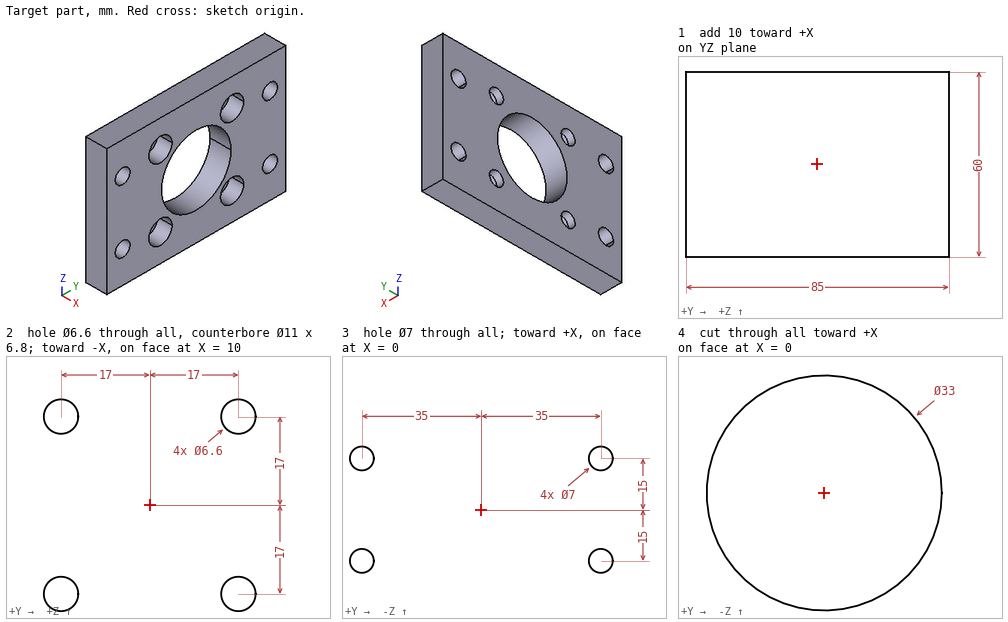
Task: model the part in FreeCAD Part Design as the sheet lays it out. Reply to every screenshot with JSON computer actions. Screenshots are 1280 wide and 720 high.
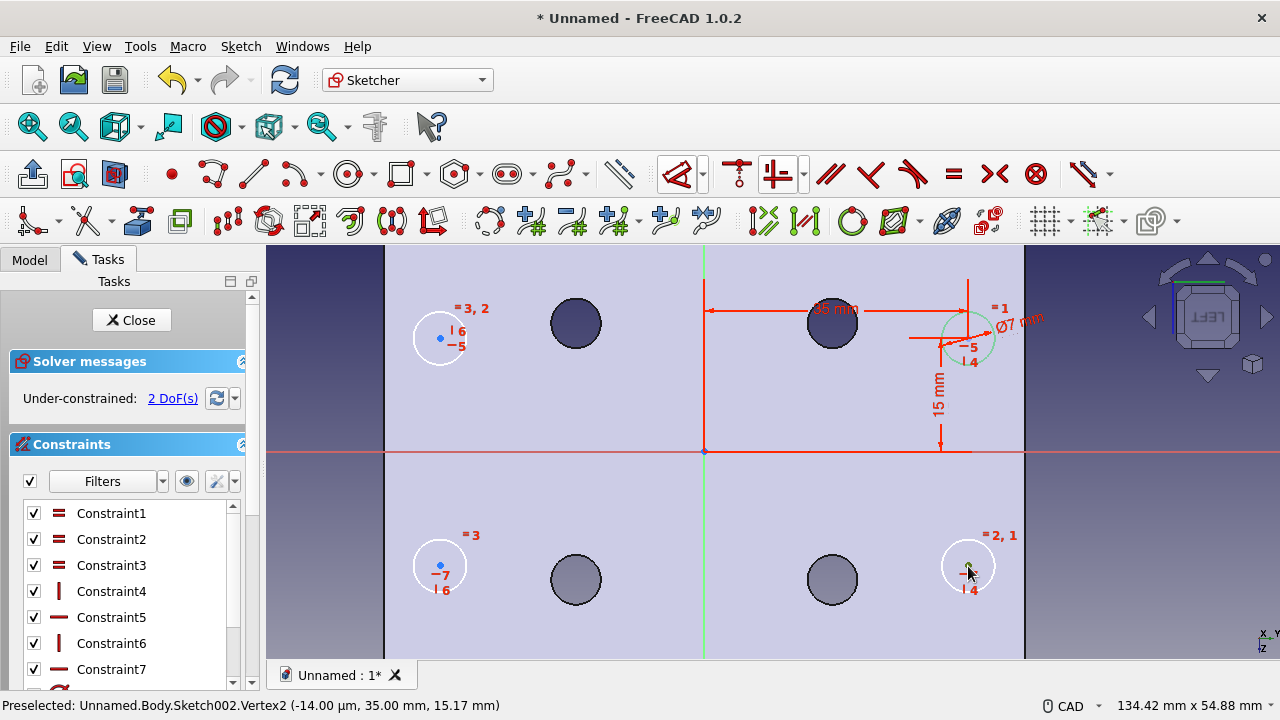
{"action": "key", "text": "i"}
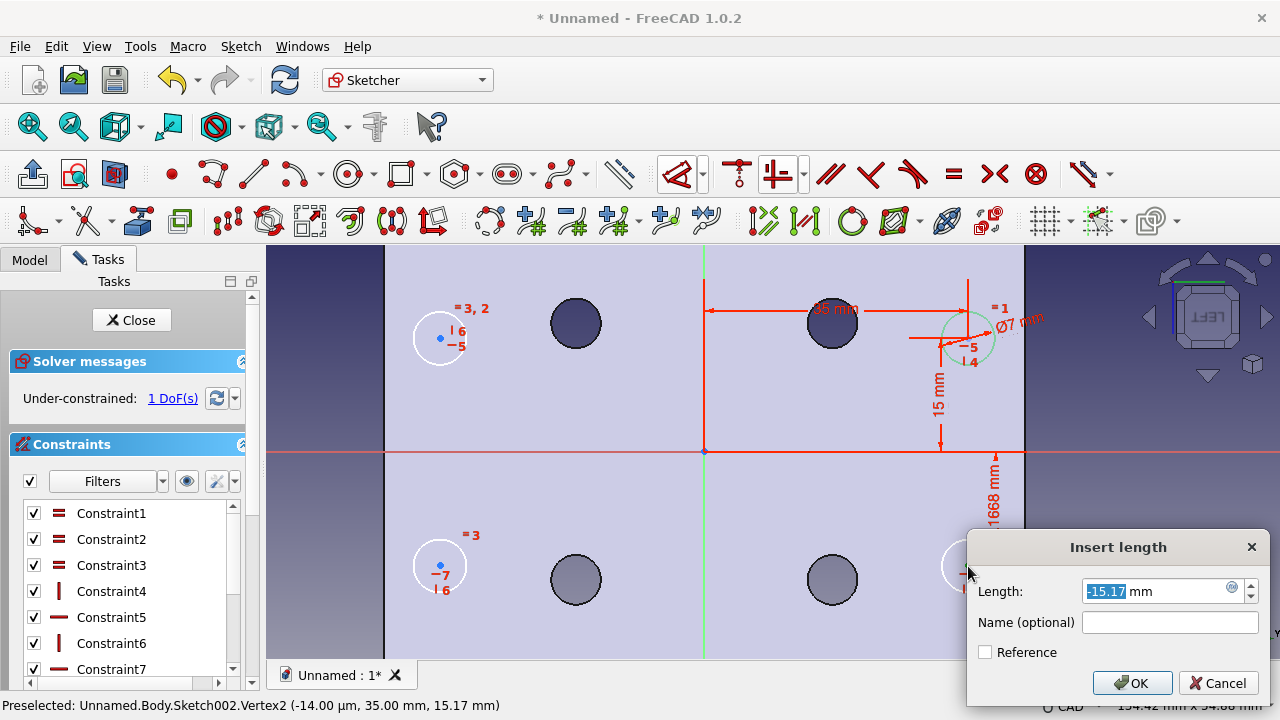
{"action": "type", "text": "-15"}
{"action": "key", "text": "Return"}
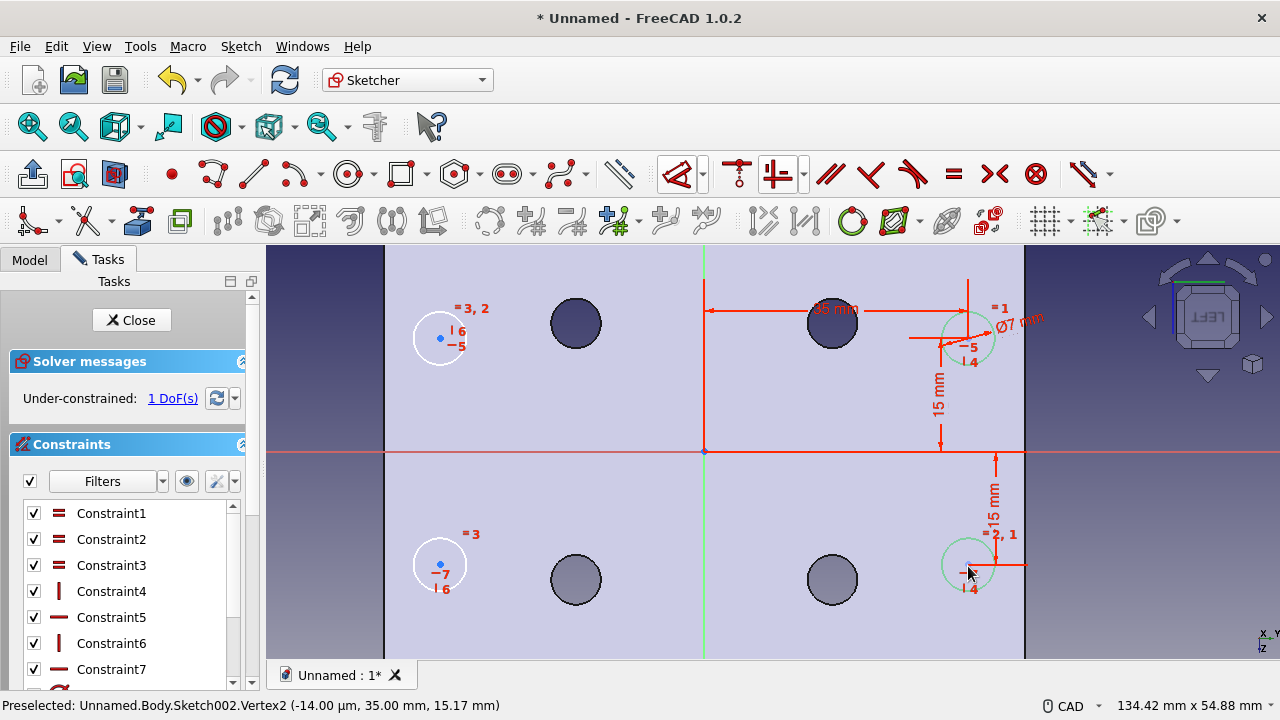
{"action": "left_click", "coordinate": [440, 338]}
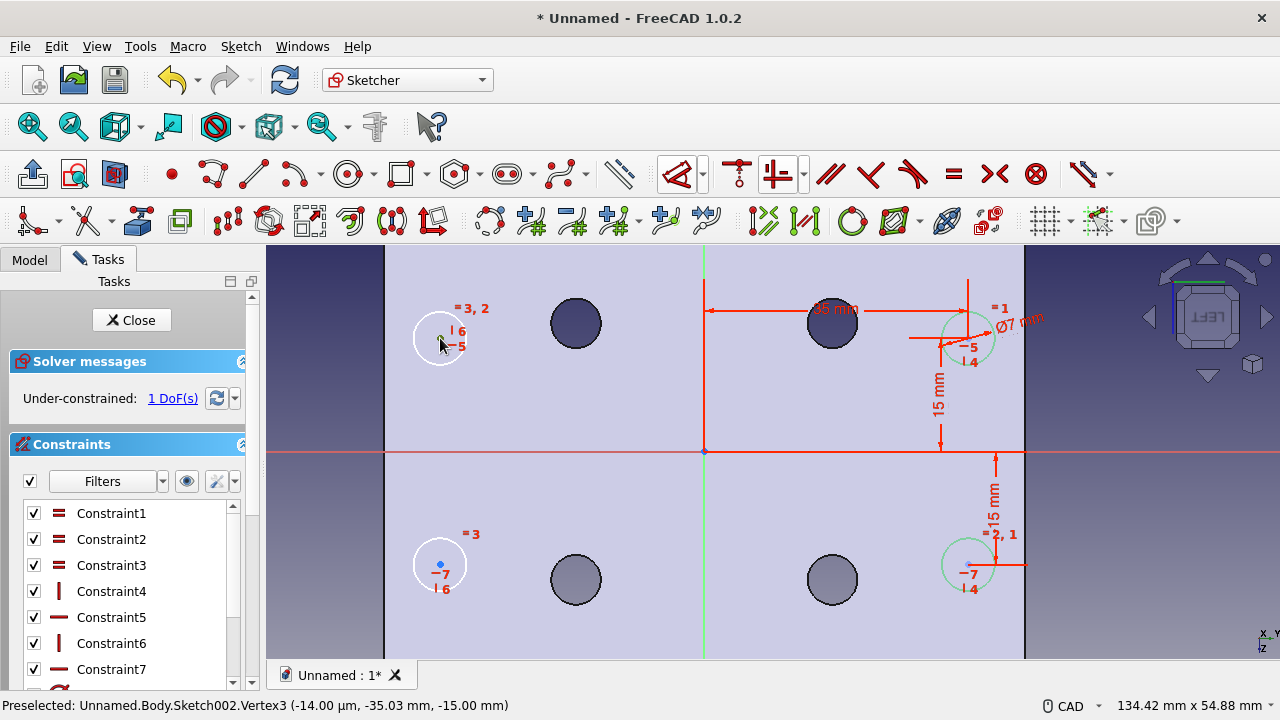
{"action": "key", "text": "l"}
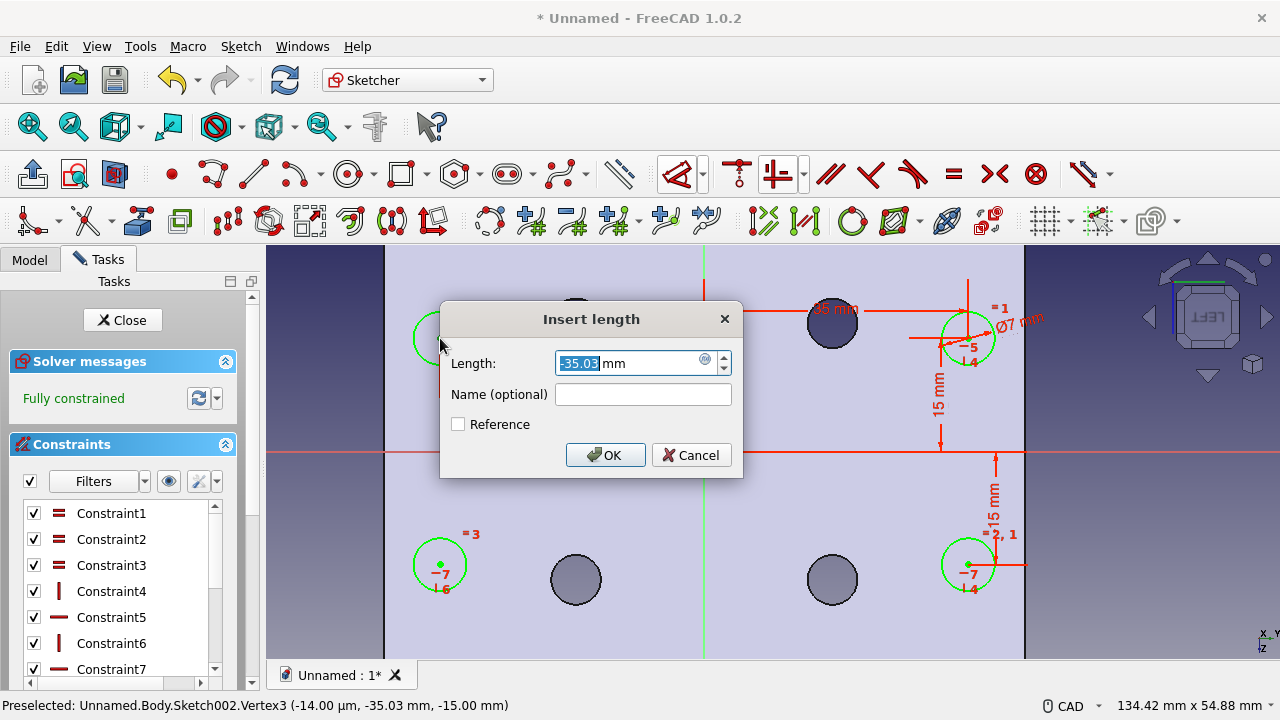
{"action": "type", "text": "-35"}
{"action": "key", "text": "Return"}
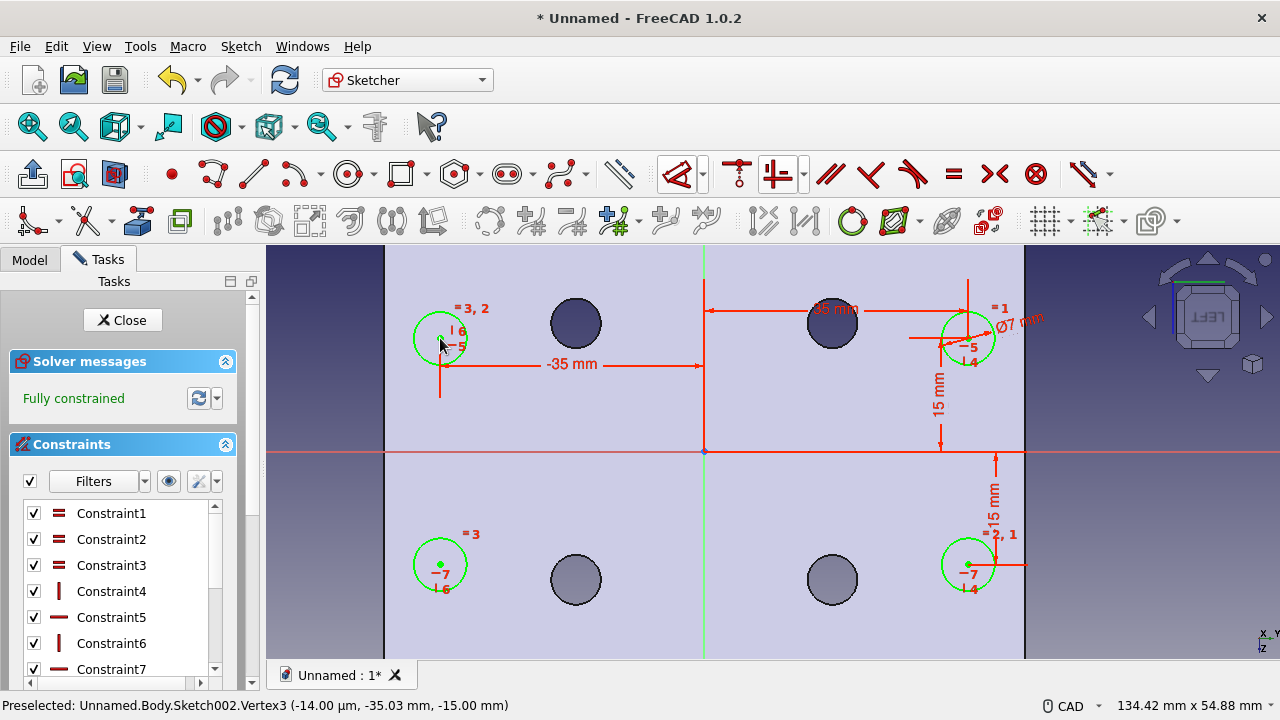
{"action": "left_click", "coordinate": [123, 320]}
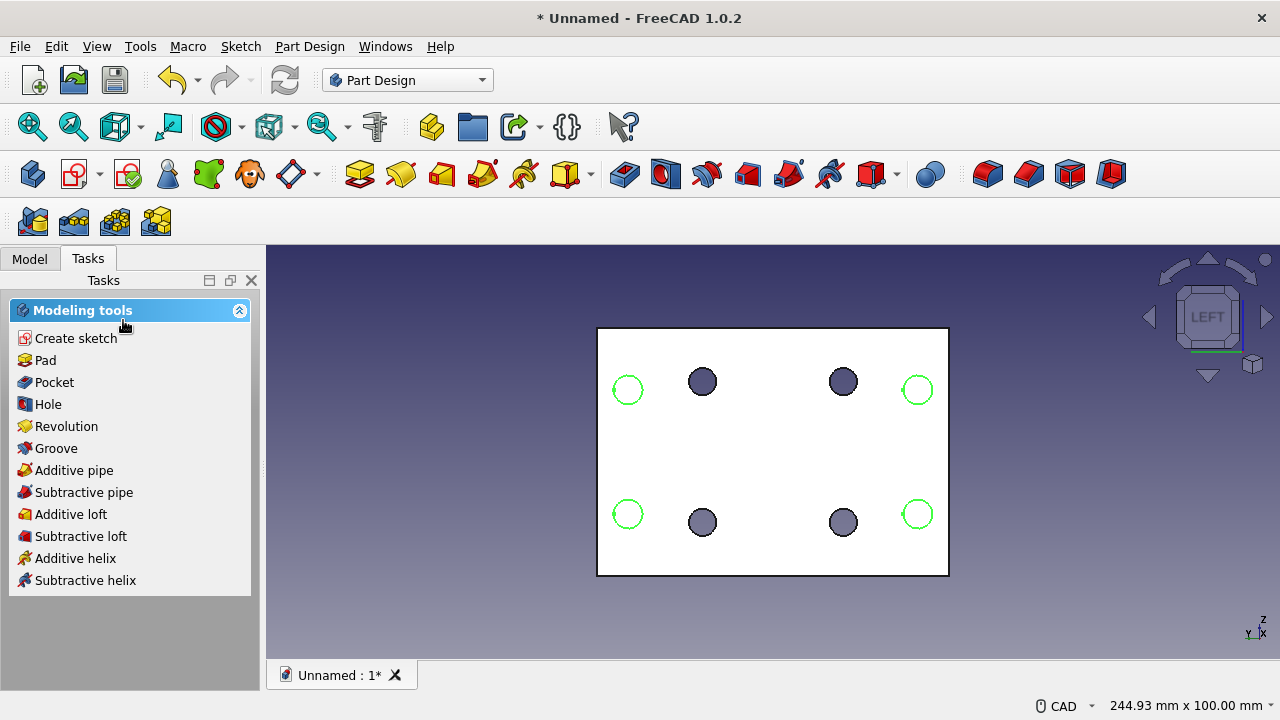
{"action": "left_click", "coordinate": [666, 174]}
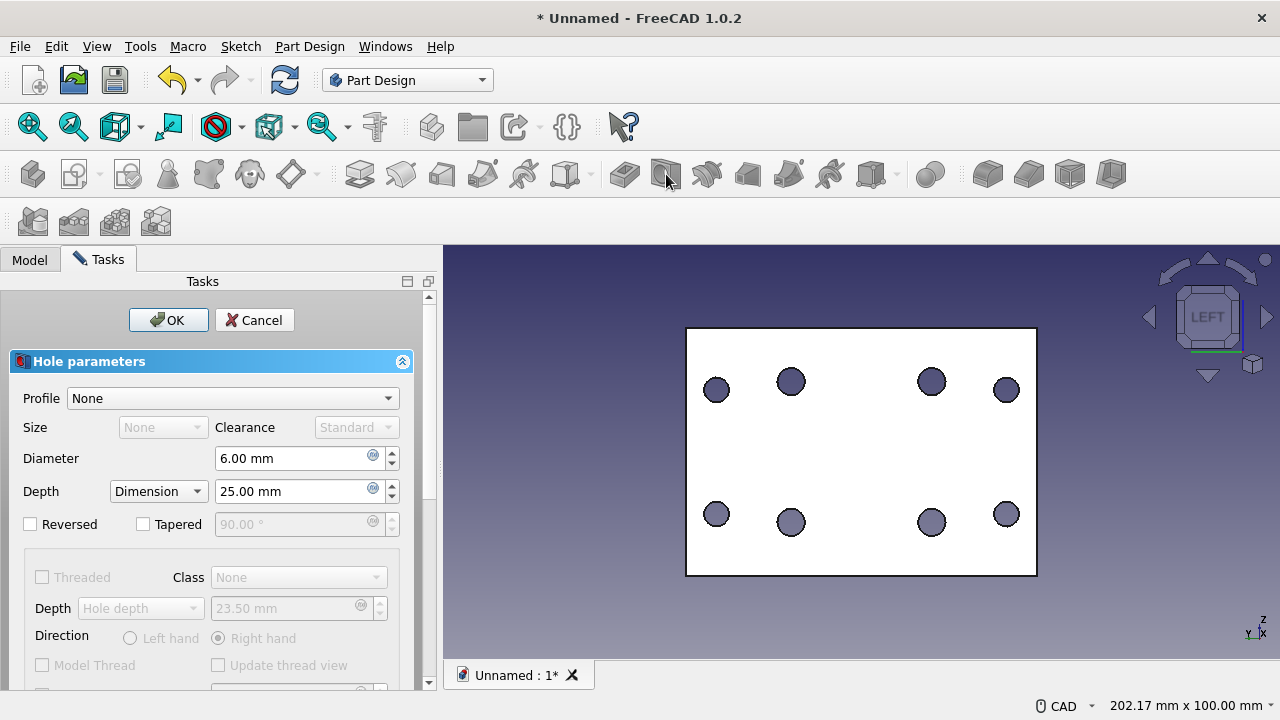
{"action": "triple_click", "coordinate": [300, 458]}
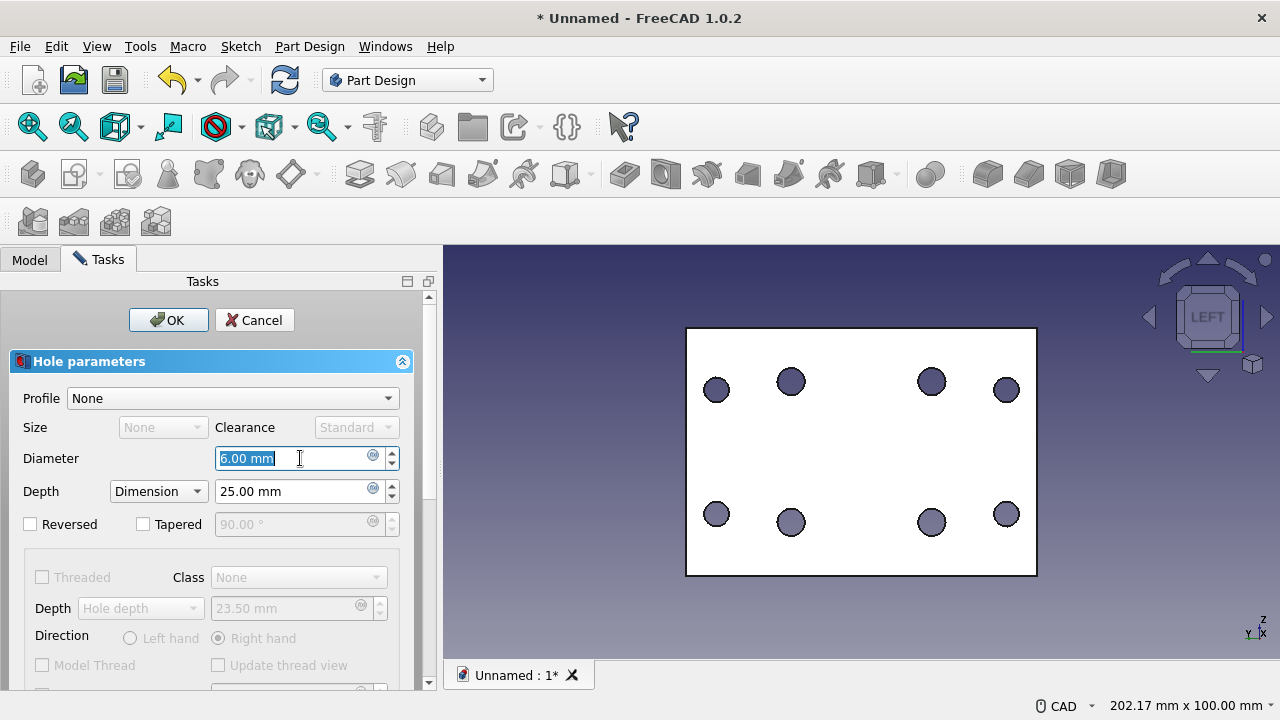
{"action": "type", "text": "7"}
{"action": "key", "text": "Tab"}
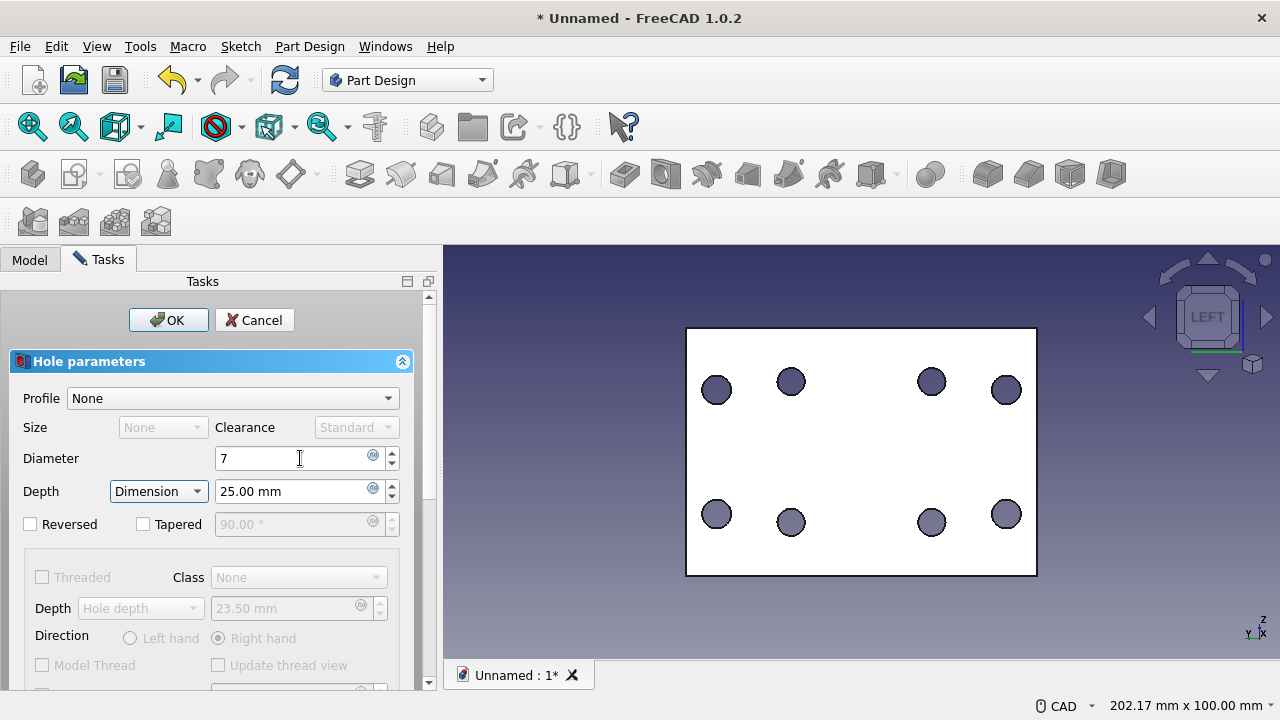
{"action": "left_click", "coordinate": [160, 492]}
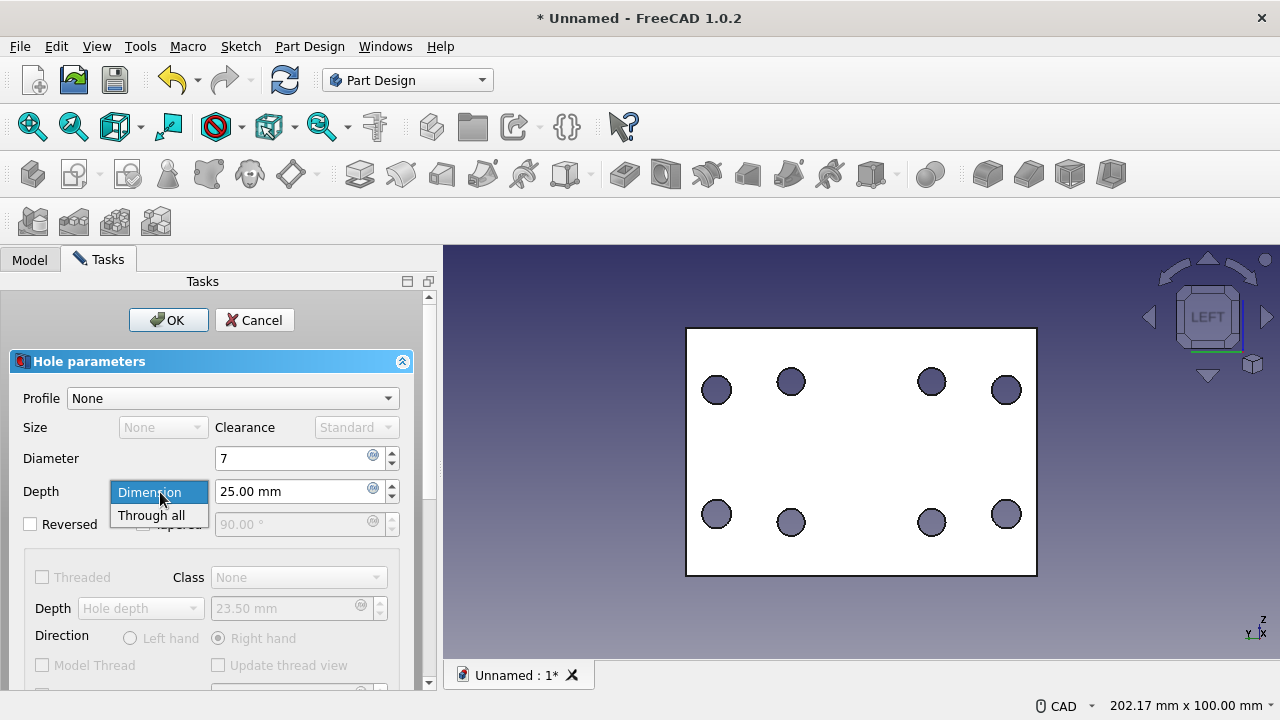
{"action": "left_click", "coordinate": [158, 516]}